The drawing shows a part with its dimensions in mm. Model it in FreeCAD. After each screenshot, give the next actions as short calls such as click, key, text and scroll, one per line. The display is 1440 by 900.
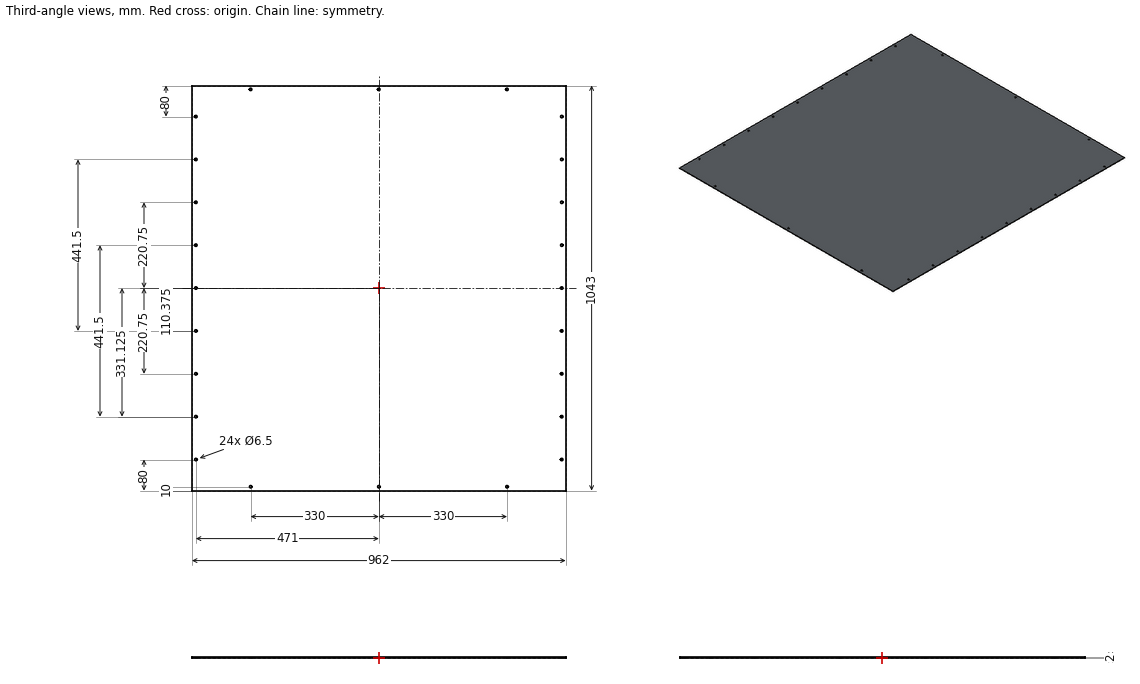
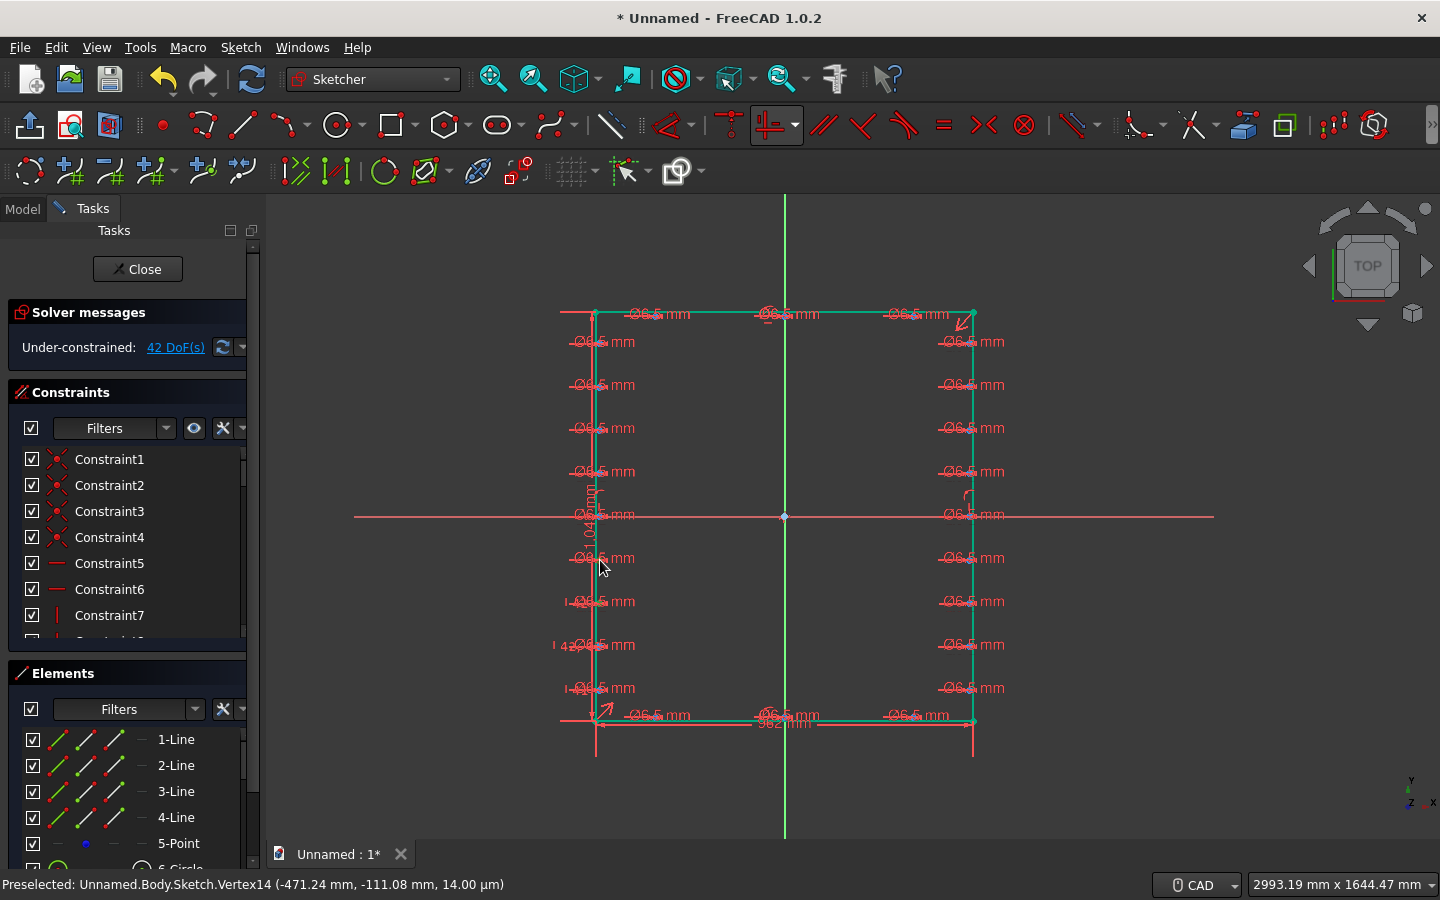
click(798, 126)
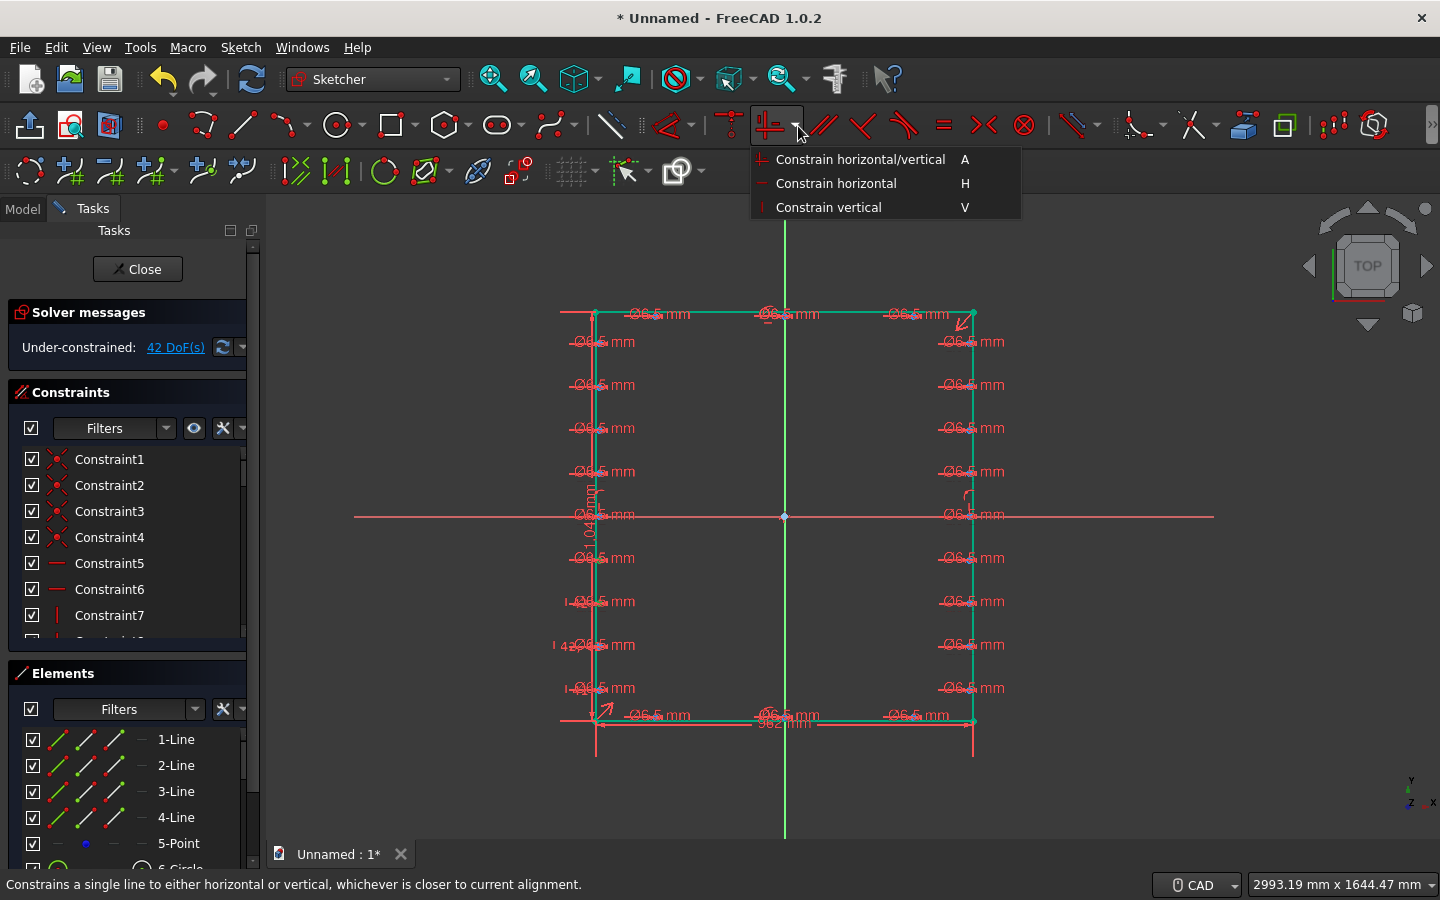
click(886, 207)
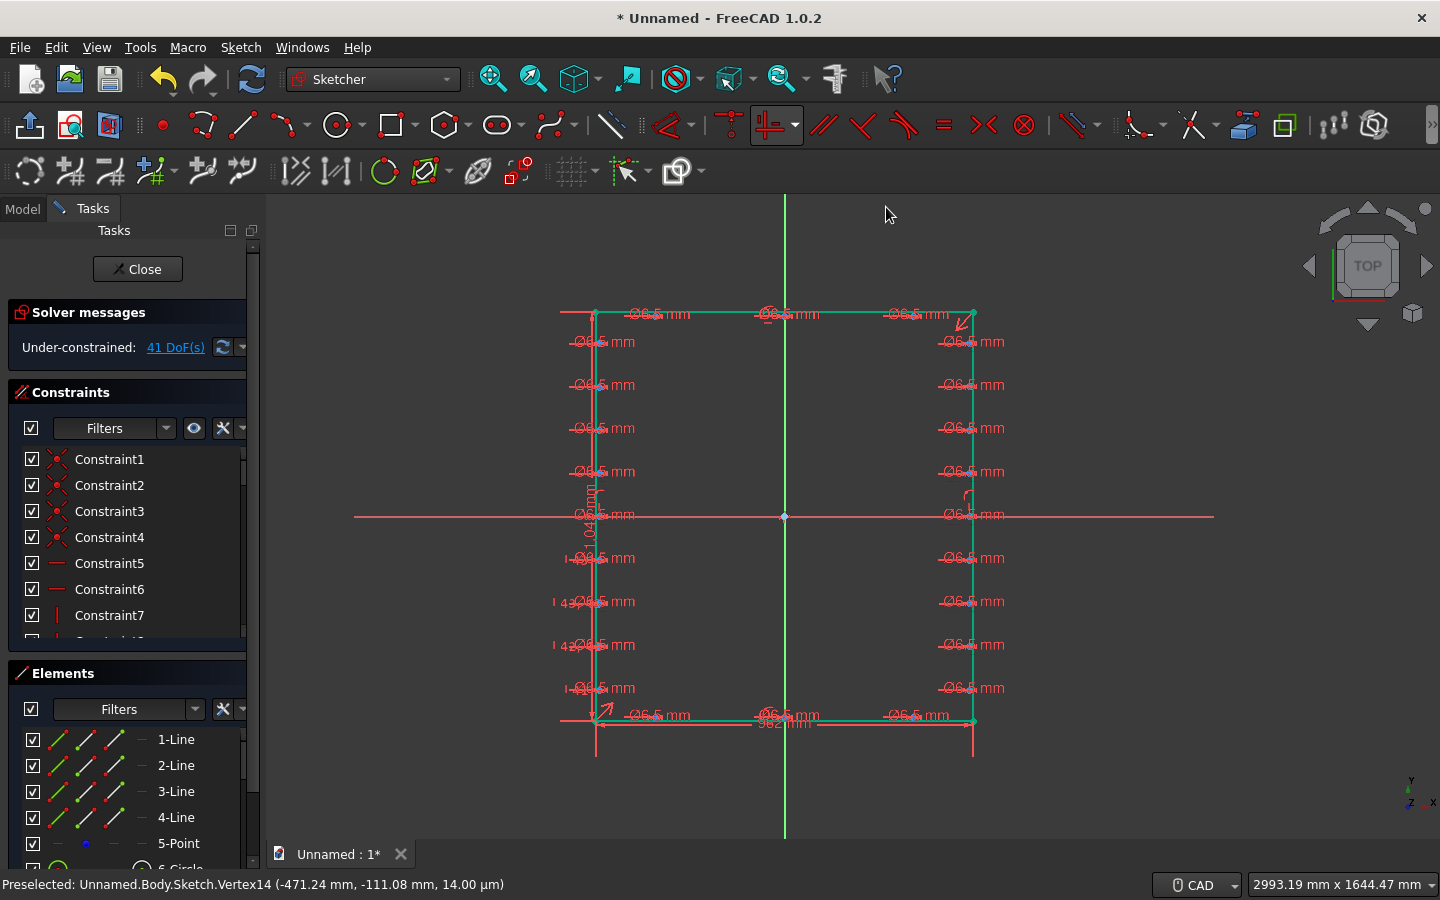
click(655, 717)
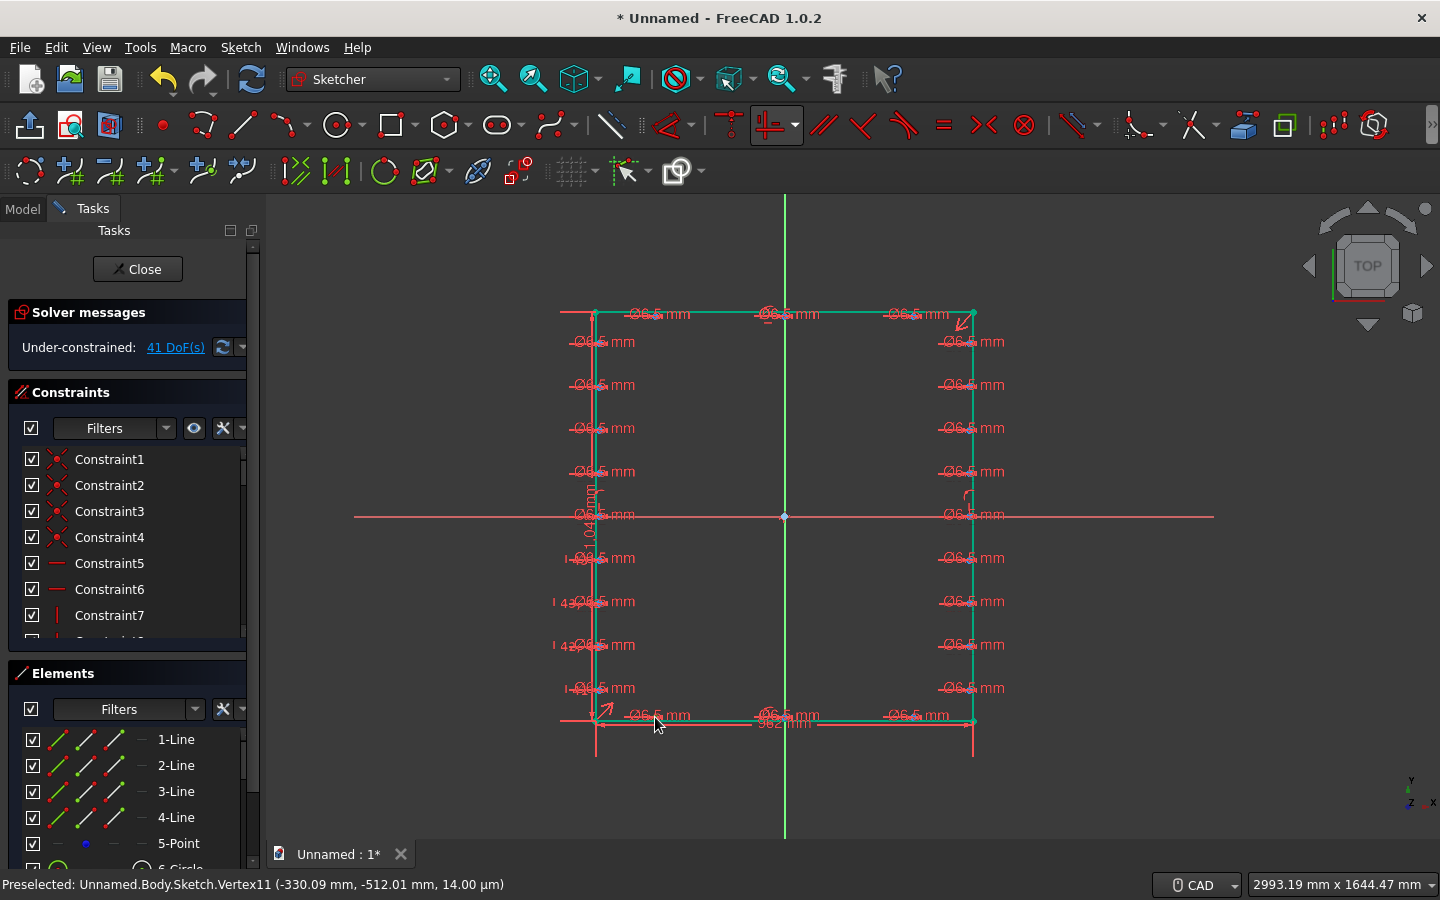
click(785, 717)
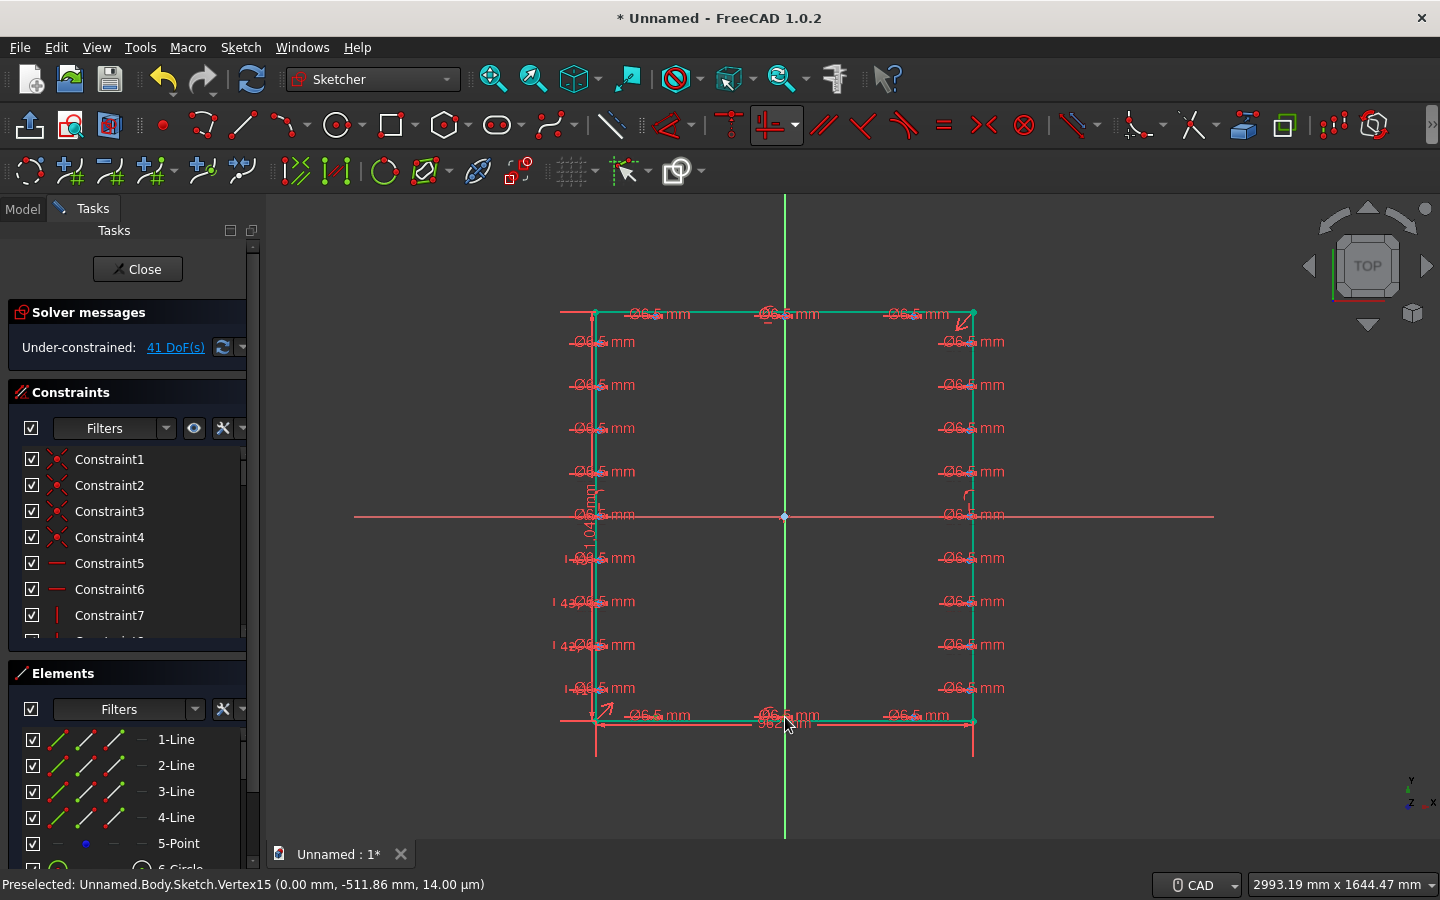
click(798, 126)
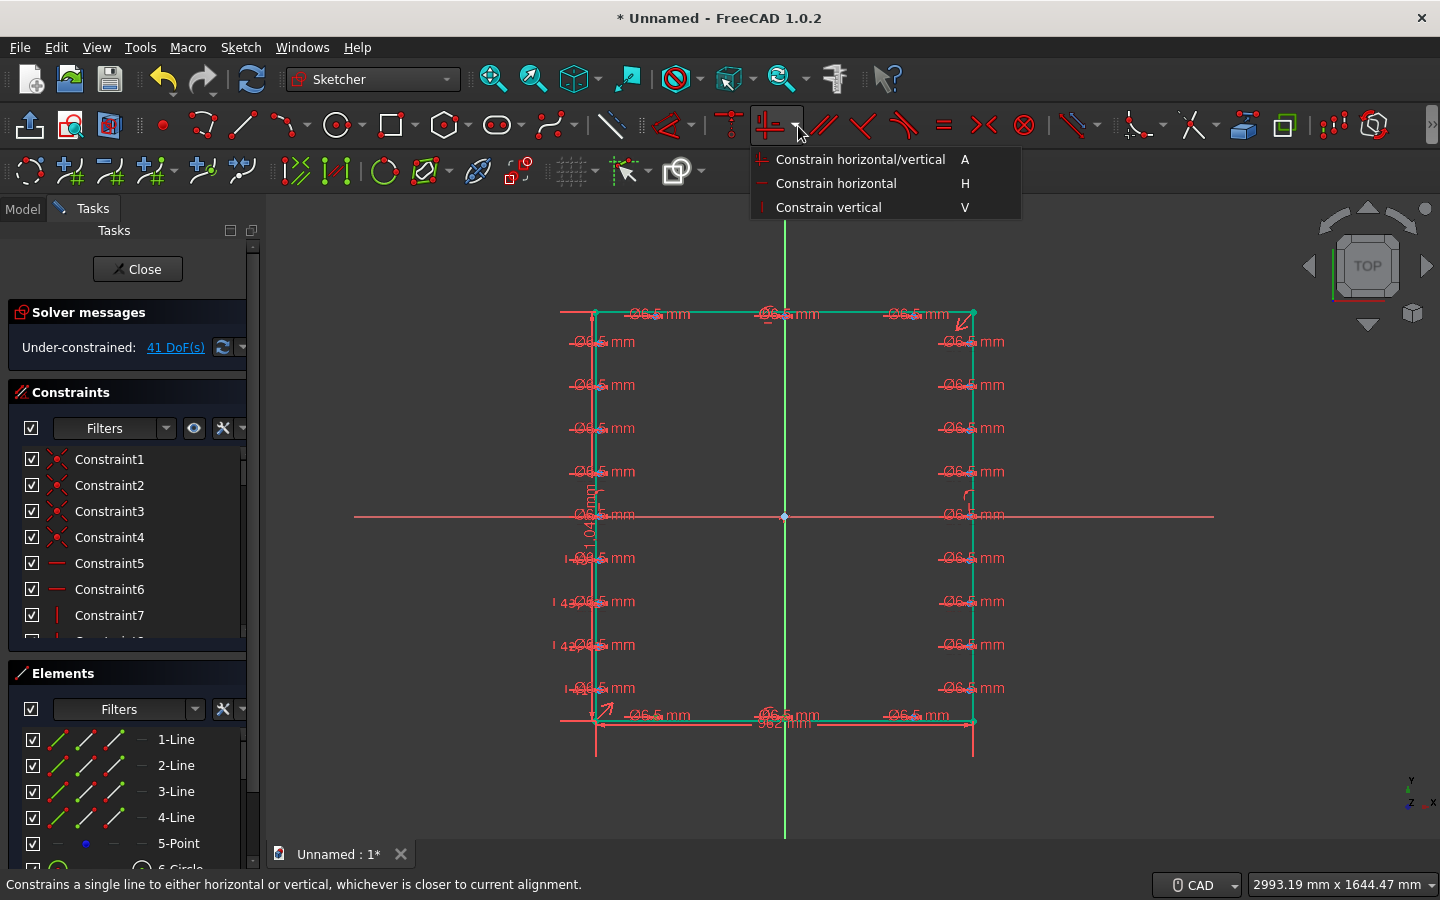
click(886, 183)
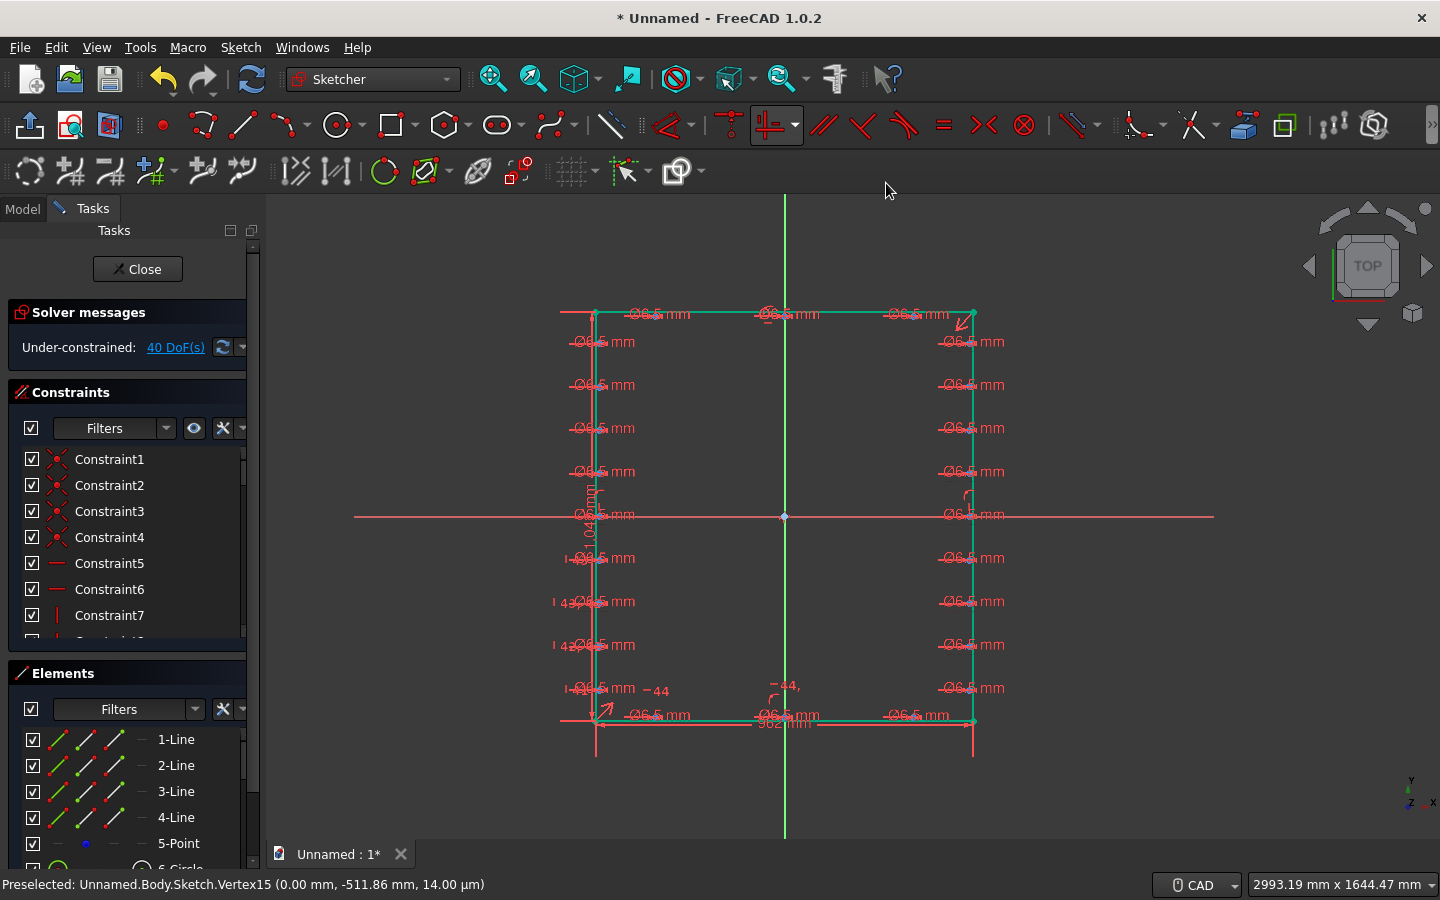
click(785, 717)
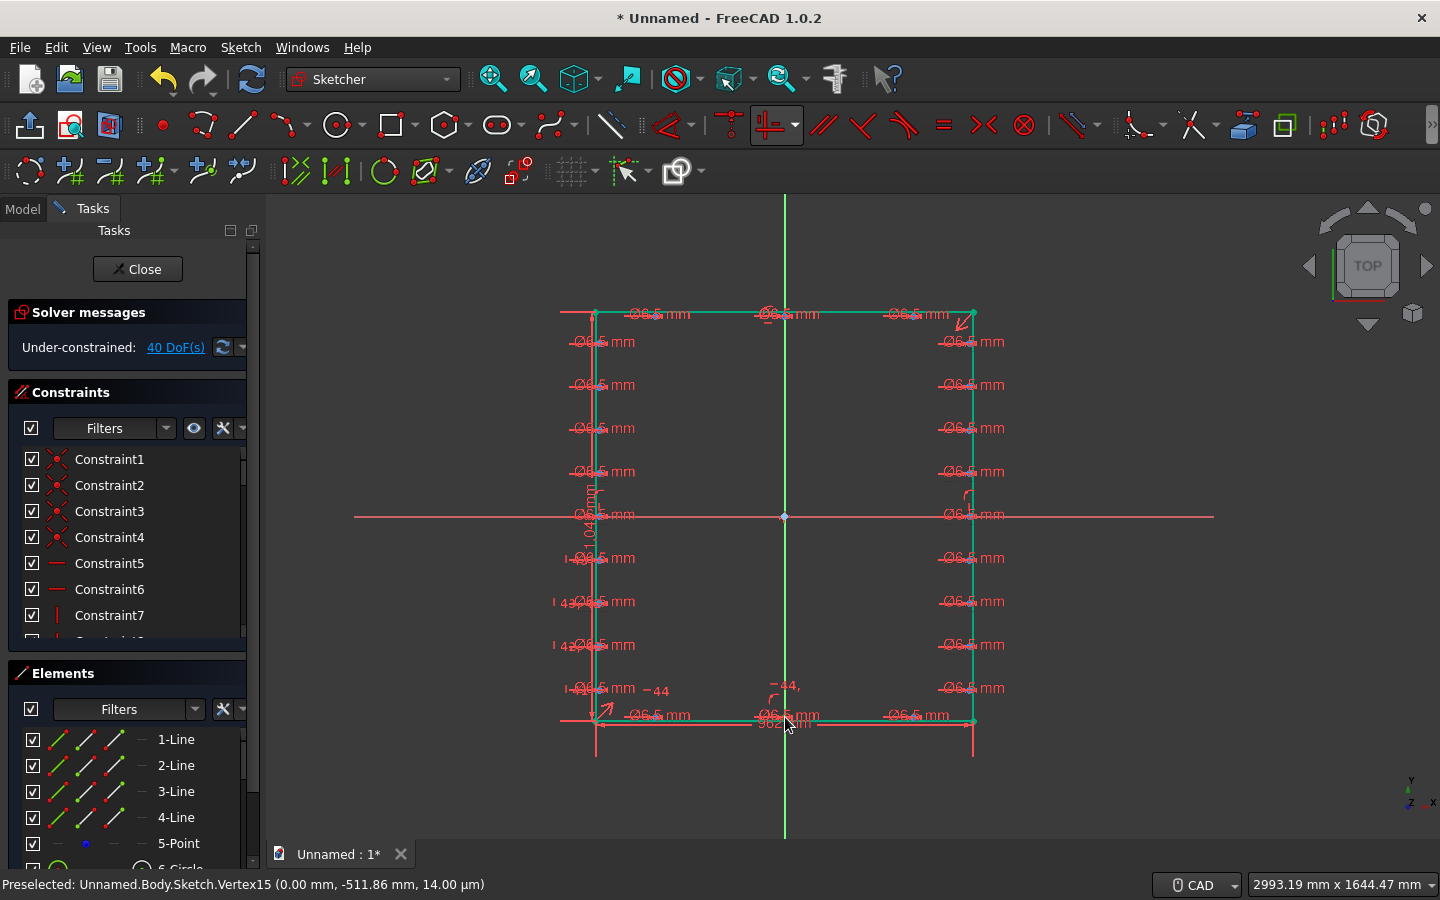
click(914, 717)